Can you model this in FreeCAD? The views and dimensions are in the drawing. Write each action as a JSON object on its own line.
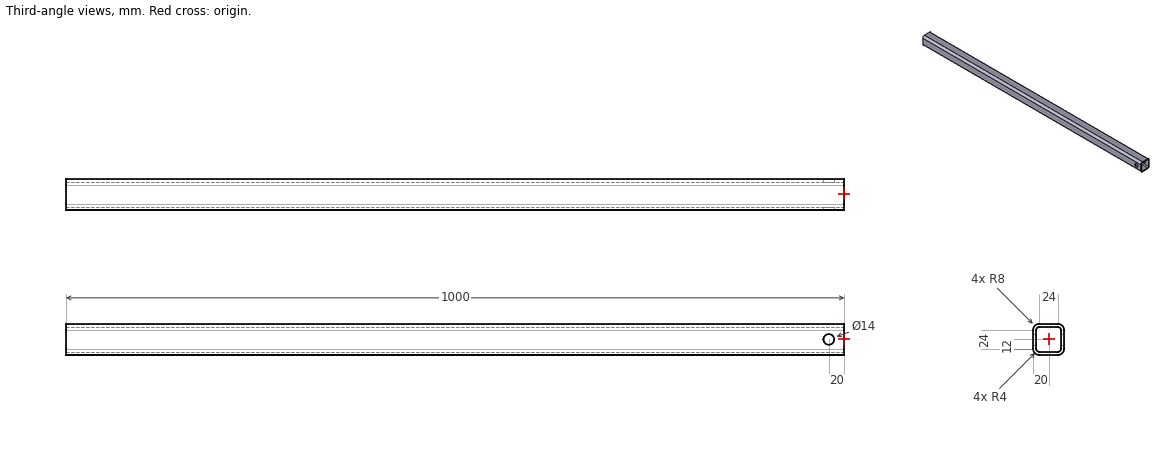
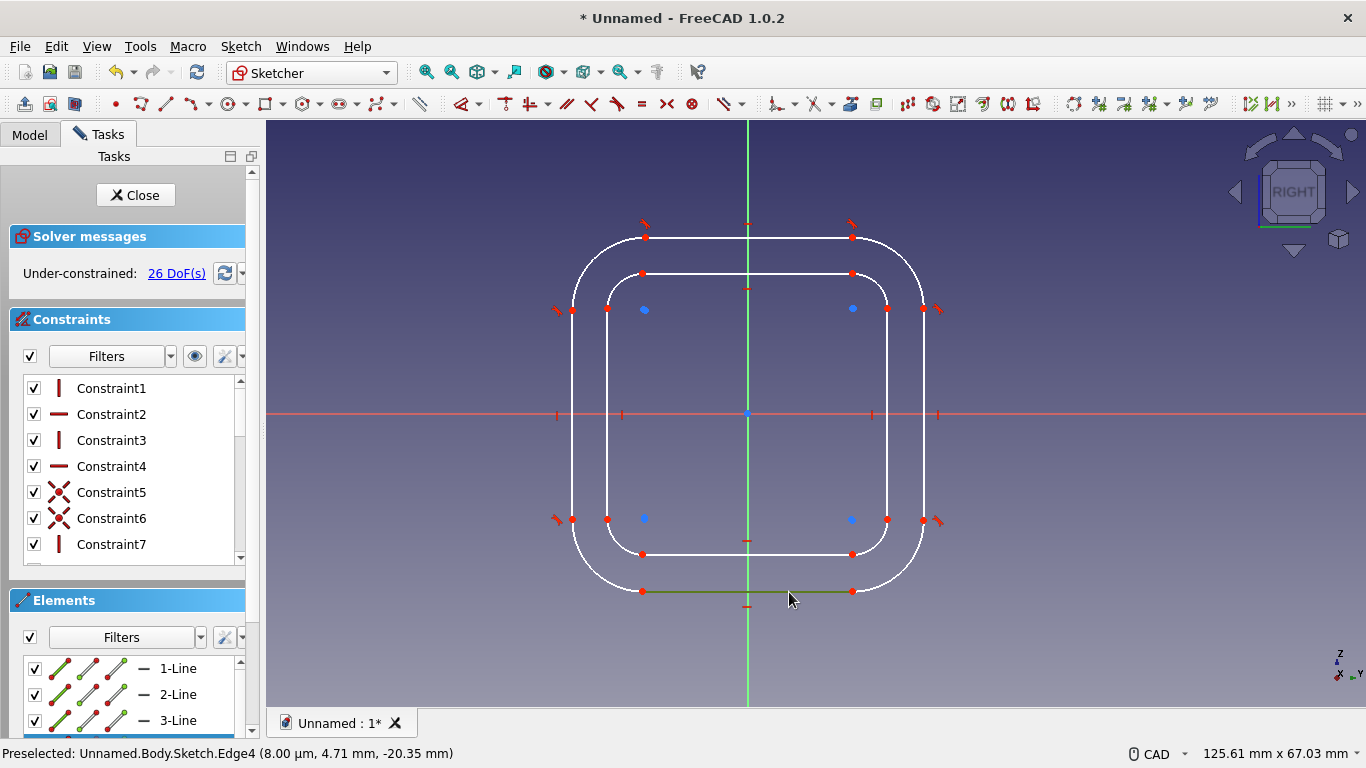
{"action": "left_click", "coordinate": [885, 584]}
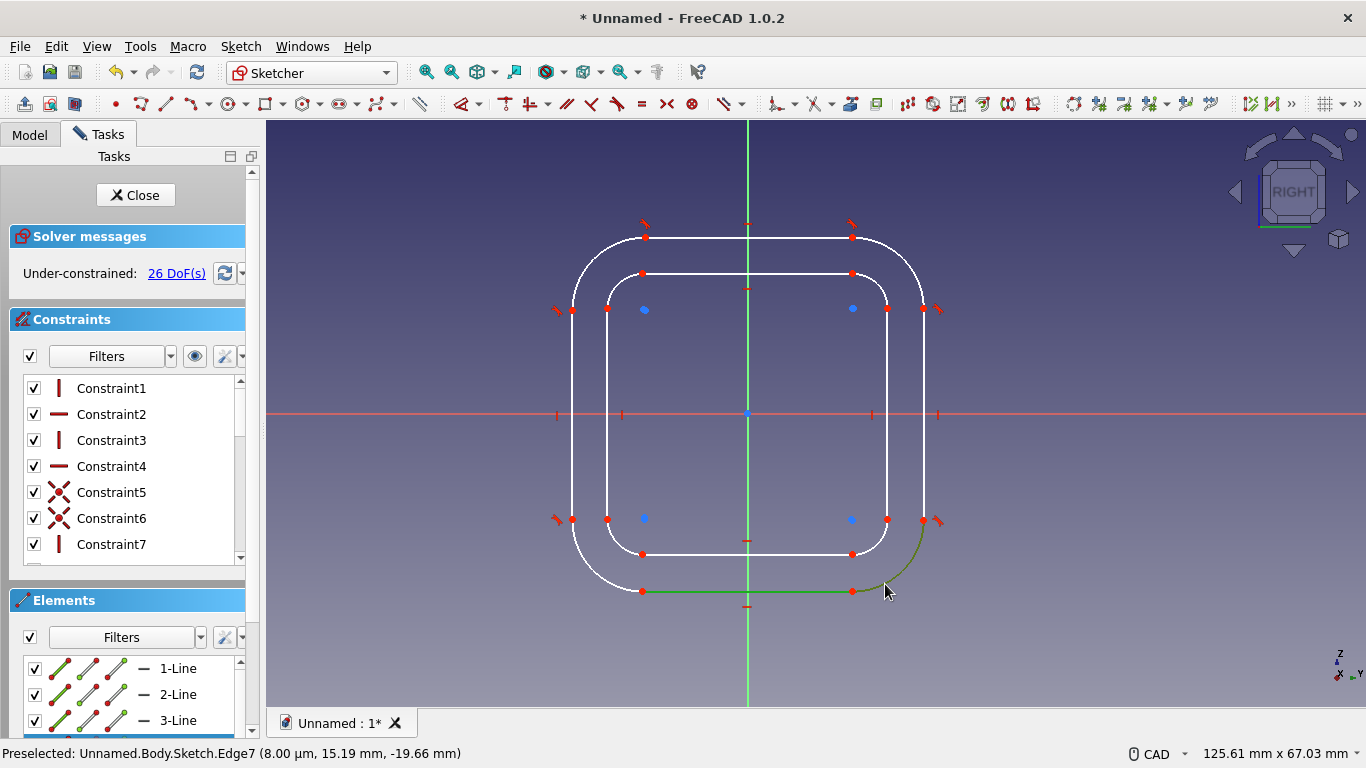
{"action": "left_click", "coordinate": [617, 104]}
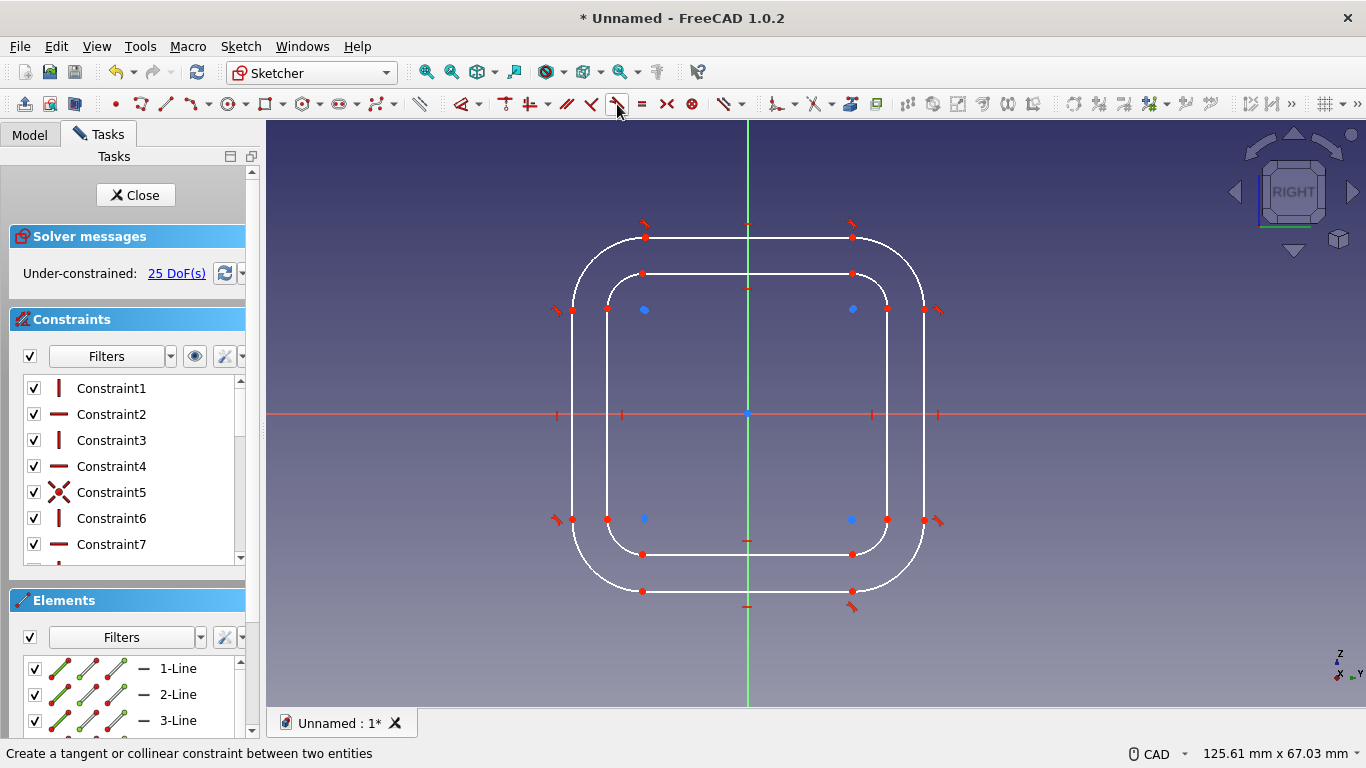
{"action": "left_click", "coordinate": [789, 592]}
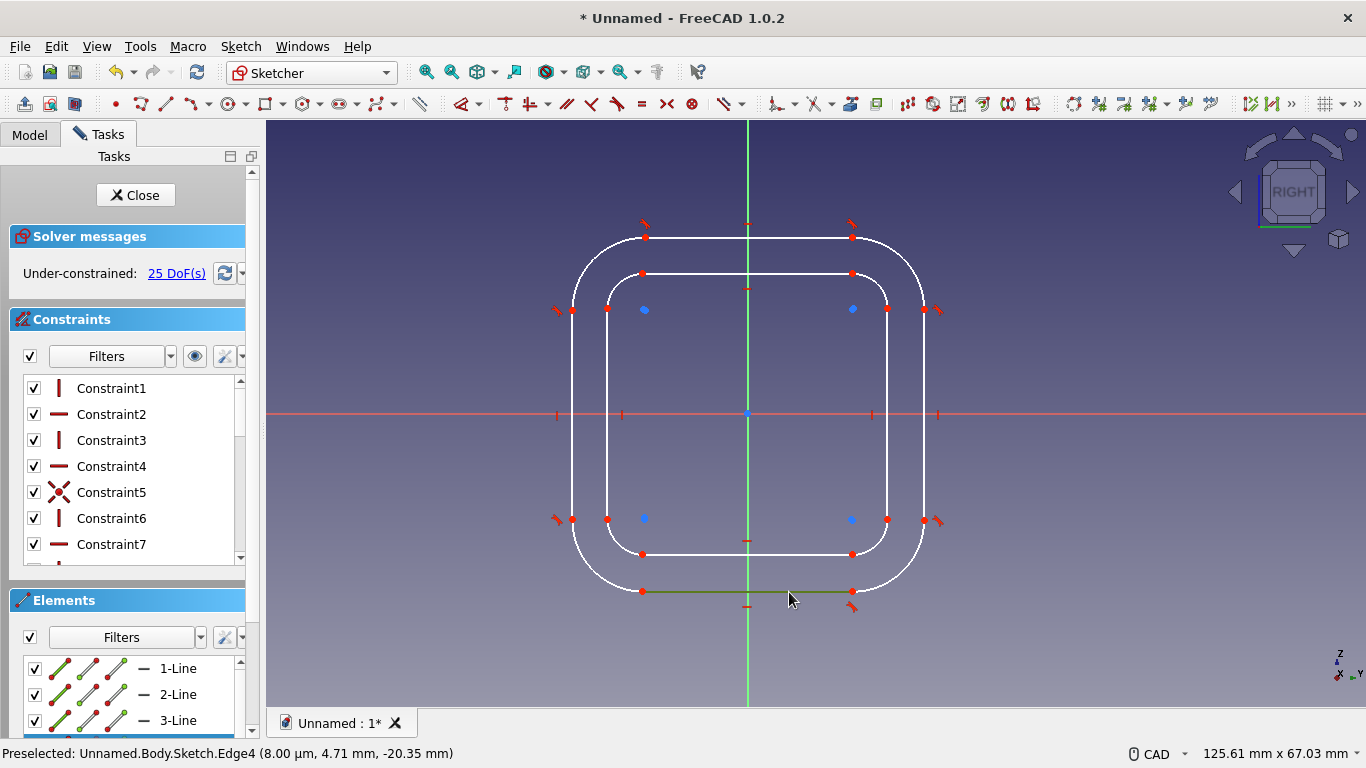
{"action": "left_click", "coordinate": [580, 552]}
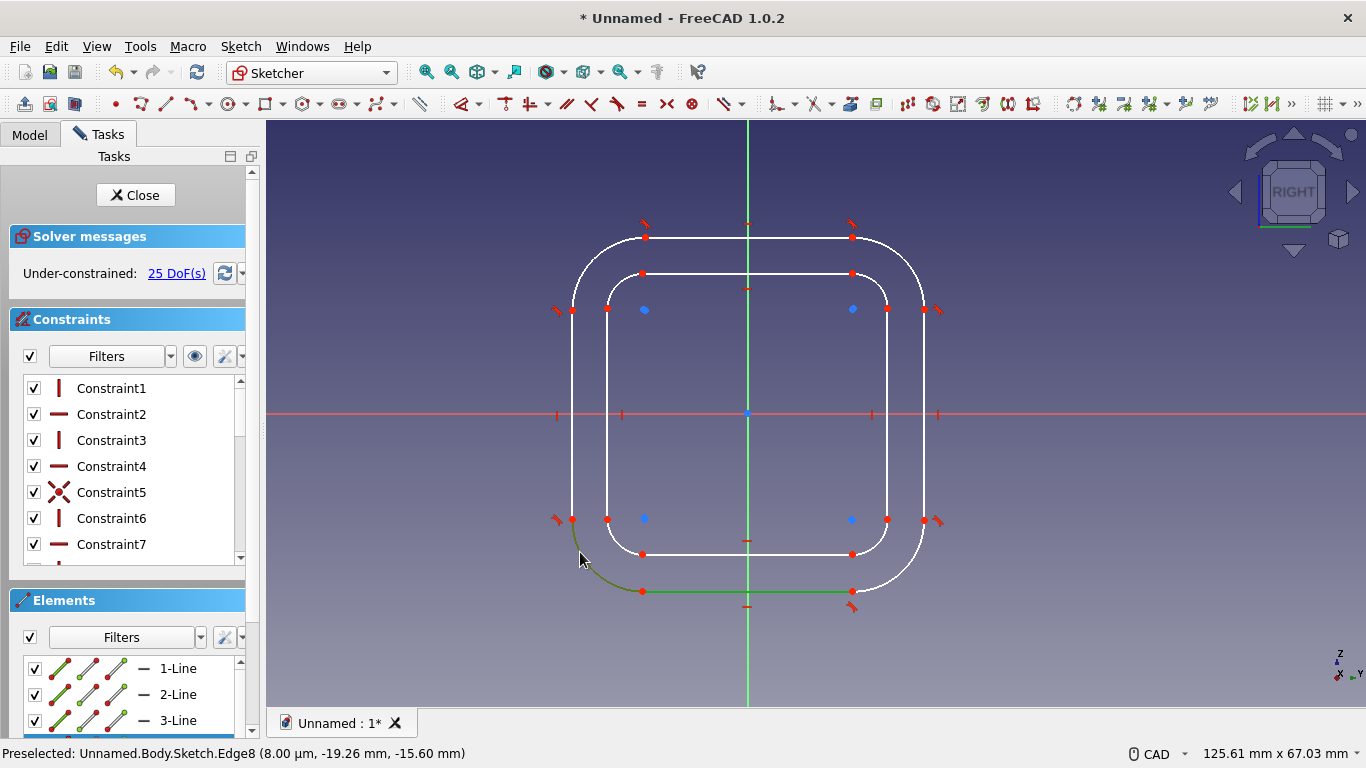
{"action": "left_click", "coordinate": [617, 104]}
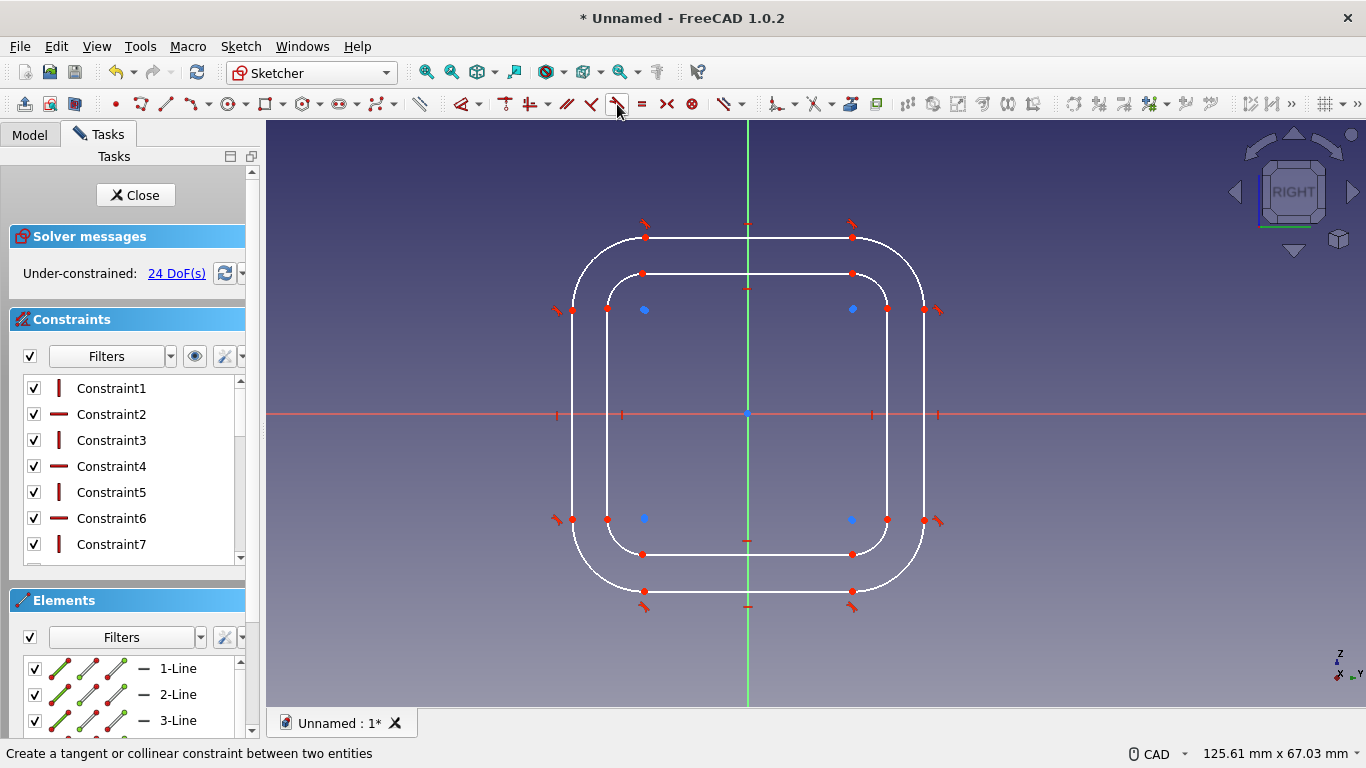
{"action": "left_click", "coordinate": [607, 372]}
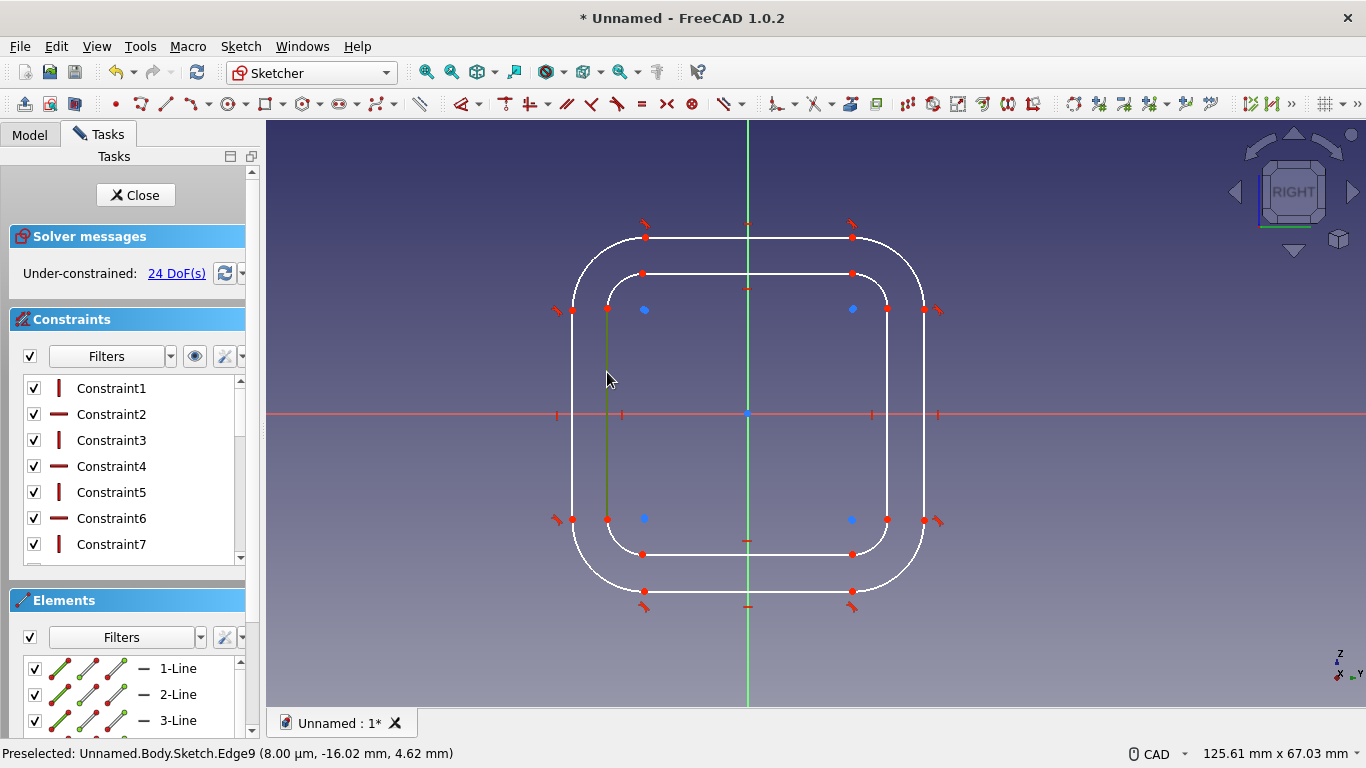
{"action": "left_click", "coordinate": [612, 535]}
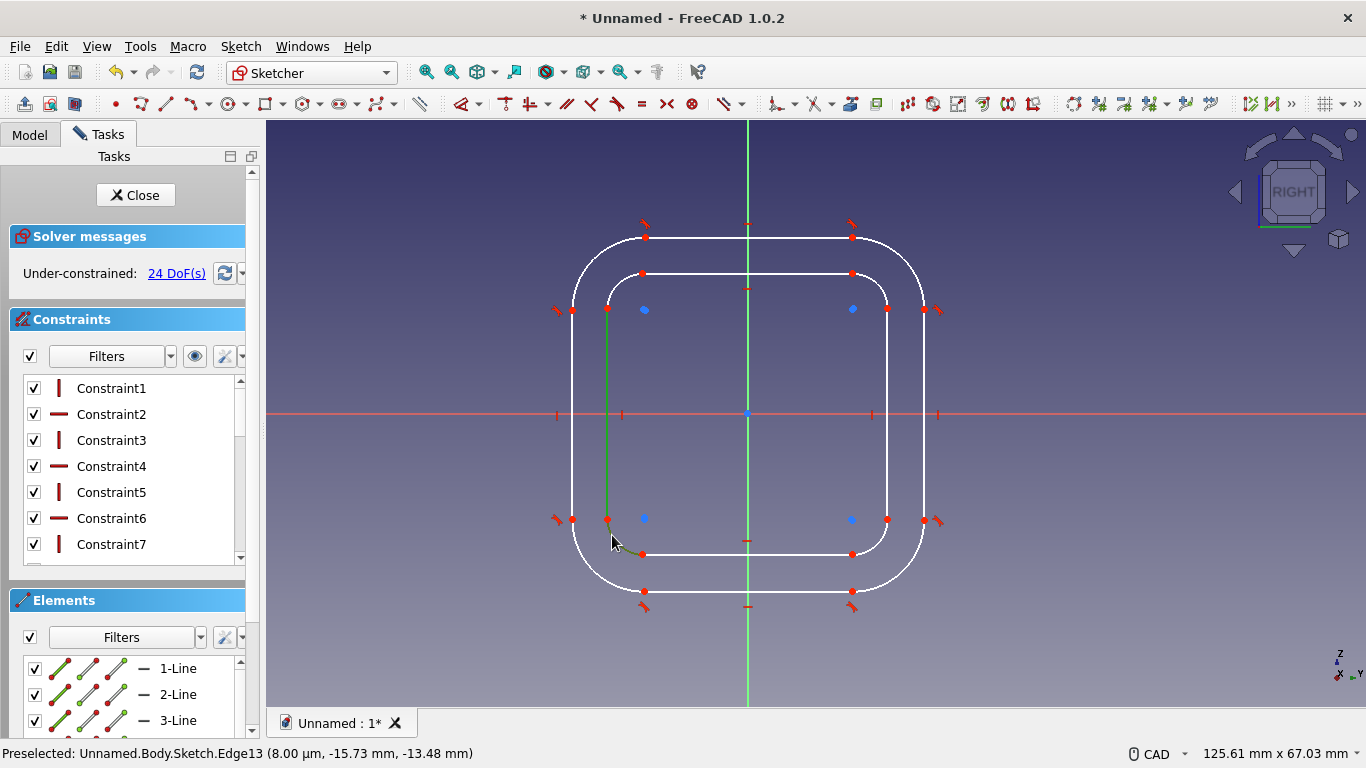
{"action": "left_click", "coordinate": [617, 104]}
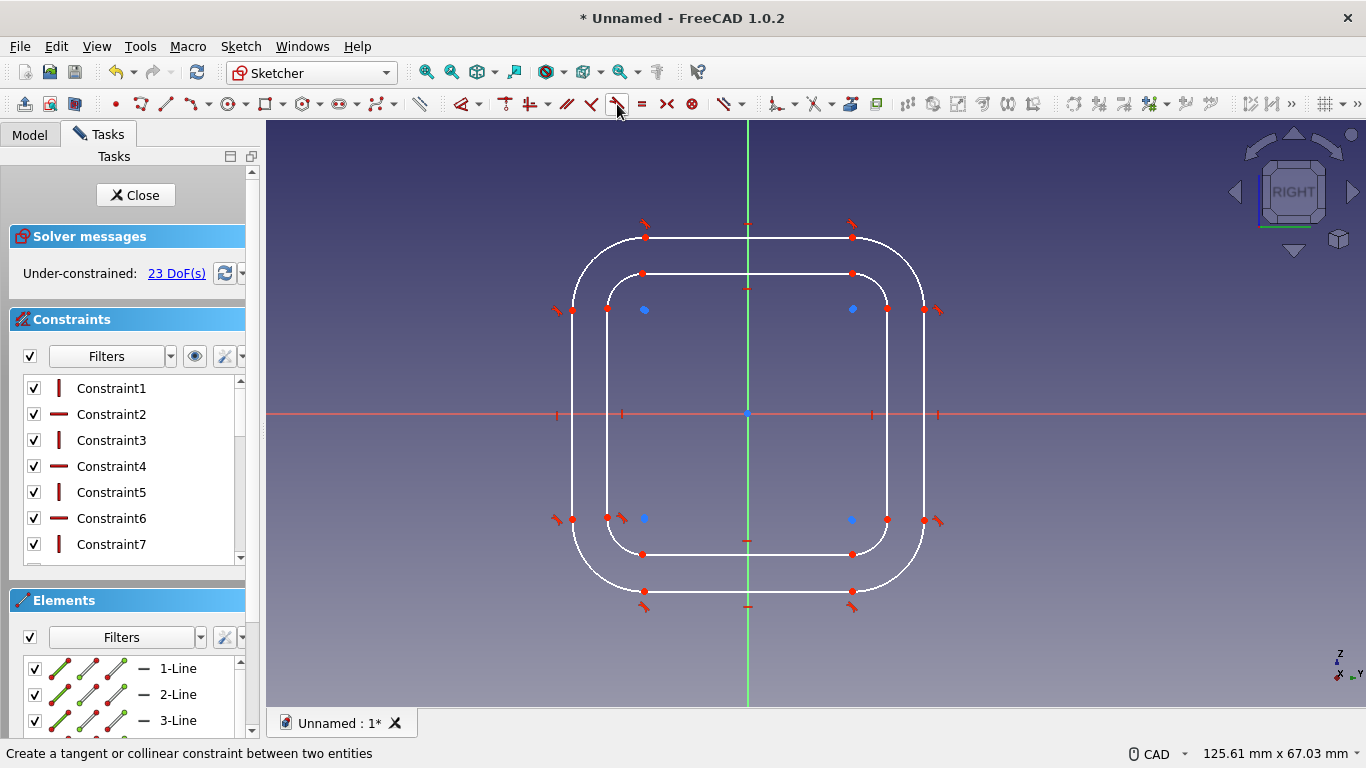
{"action": "left_click", "coordinate": [607, 372]}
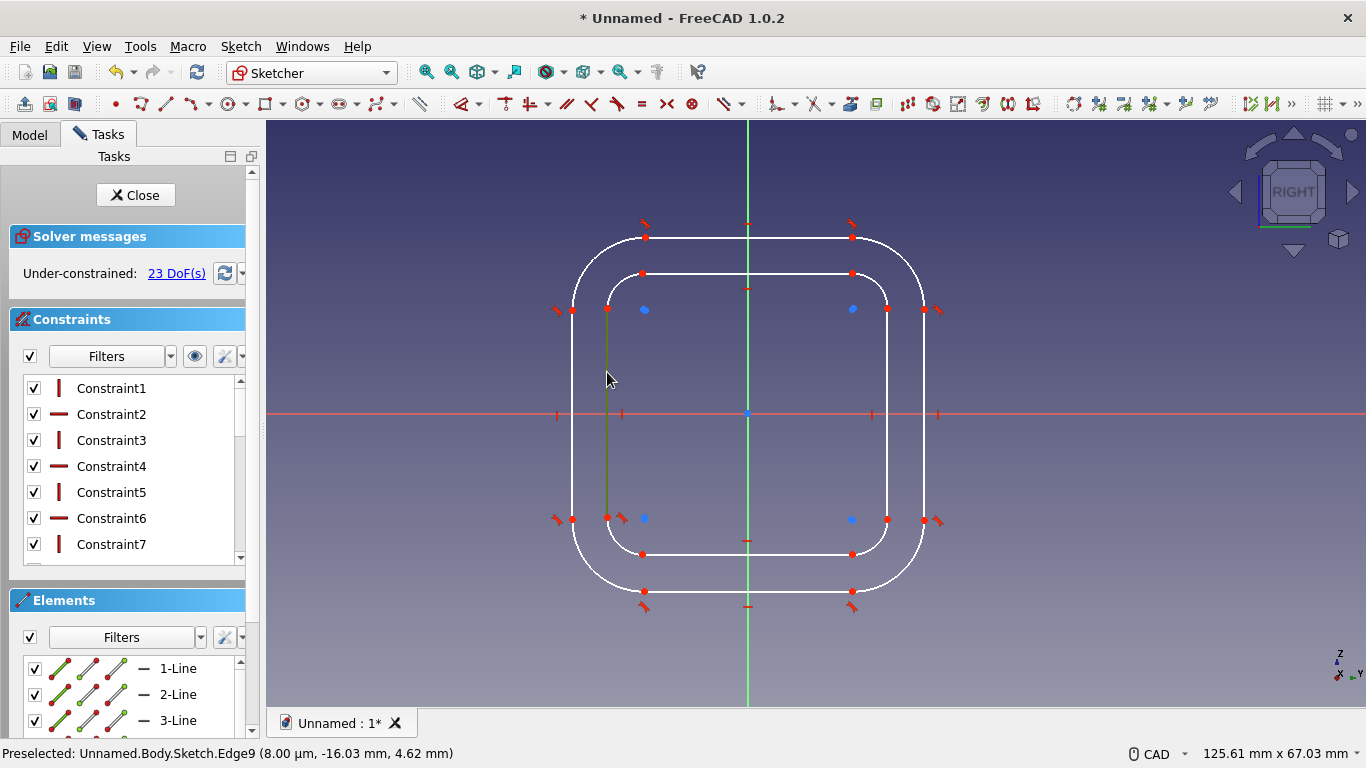
{"action": "left_click", "coordinate": [627, 278]}